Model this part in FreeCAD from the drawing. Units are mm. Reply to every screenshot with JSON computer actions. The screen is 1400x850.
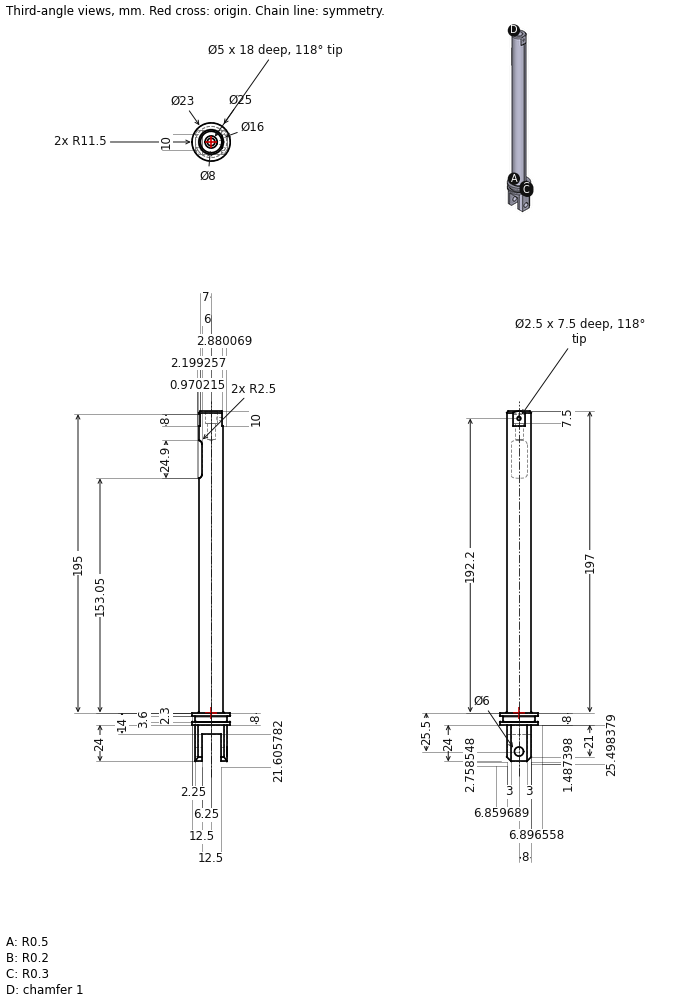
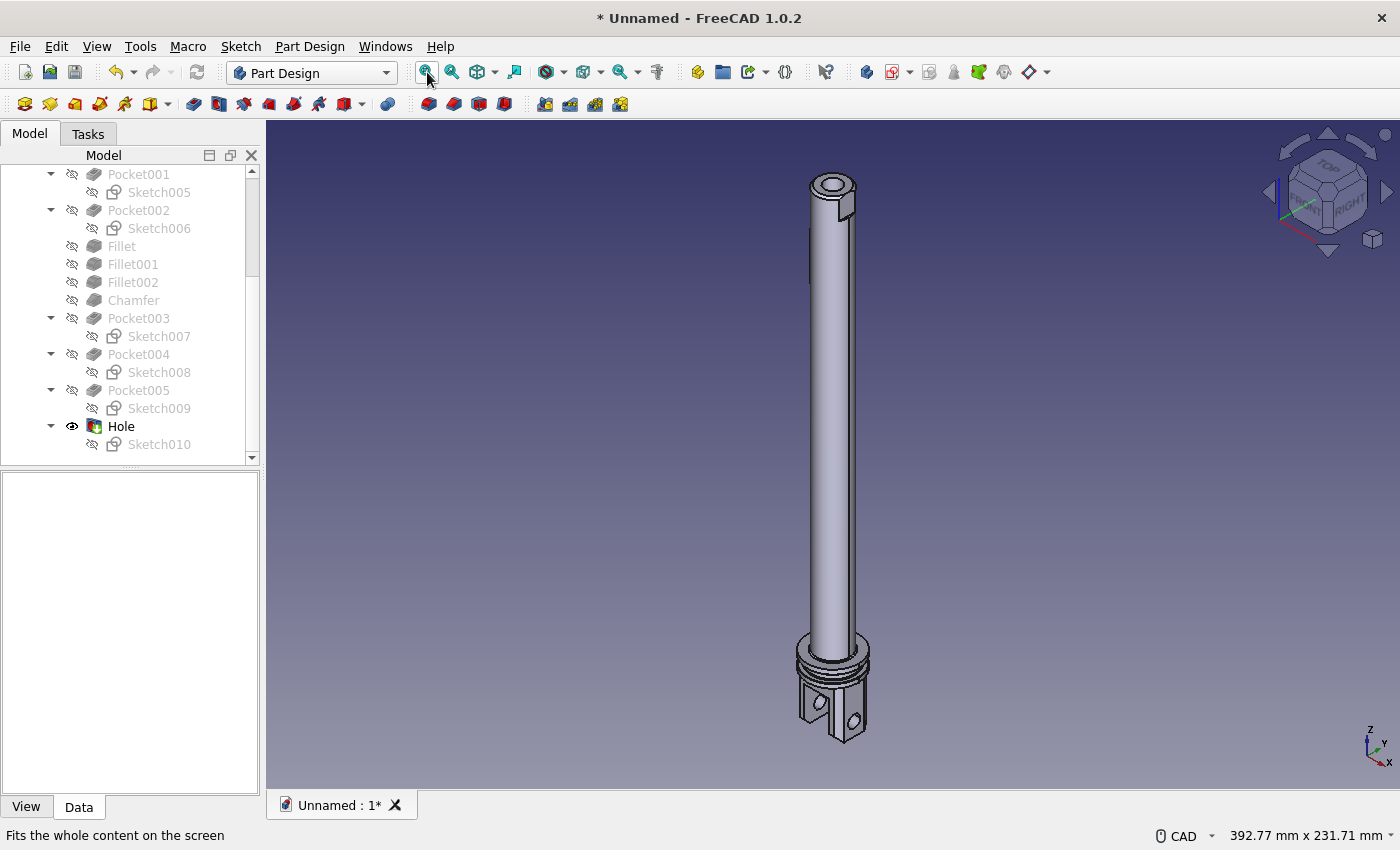
{"action": "left_click", "coordinate": [850, 202]}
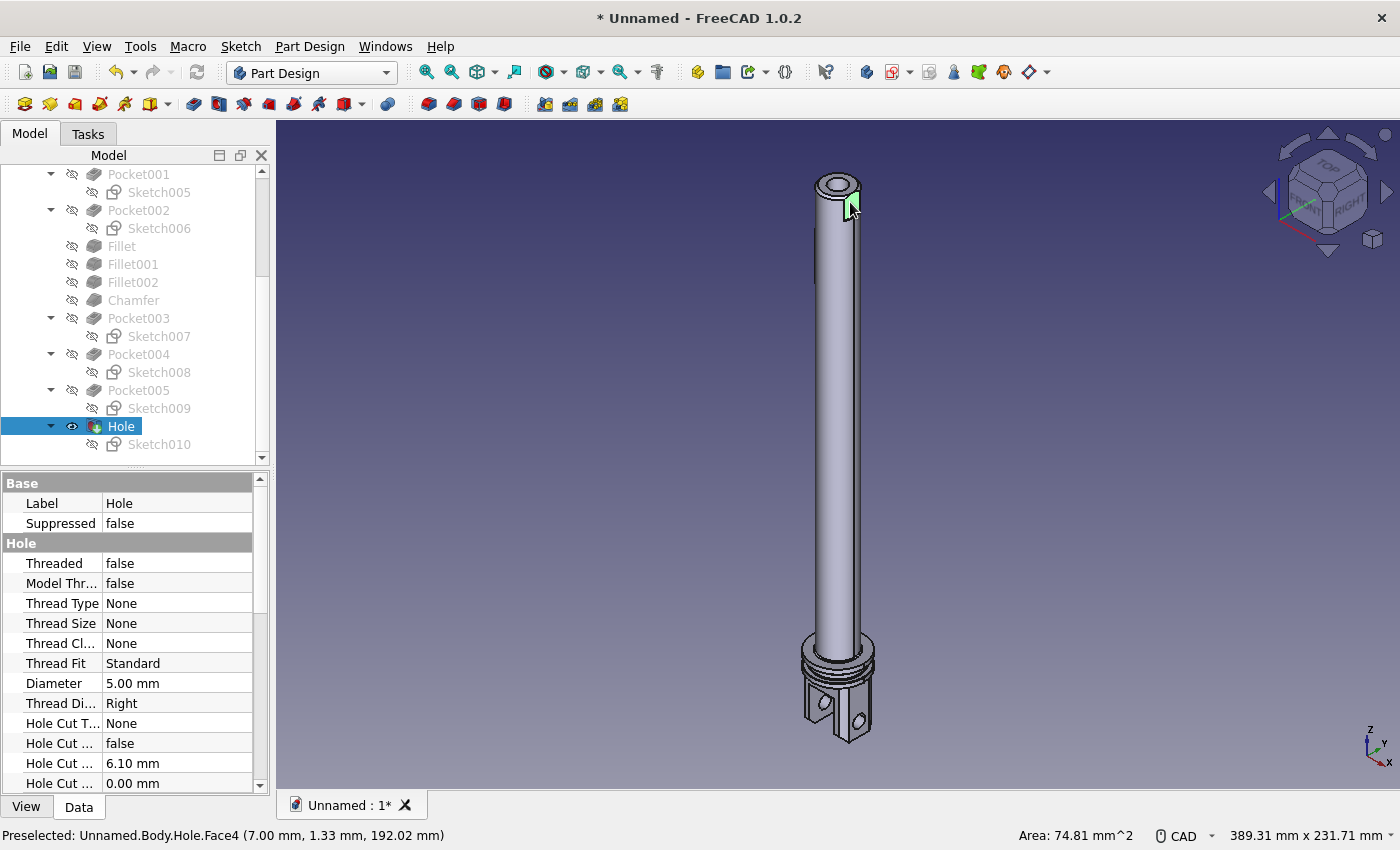
{"action": "left_click", "coordinate": [892, 72]}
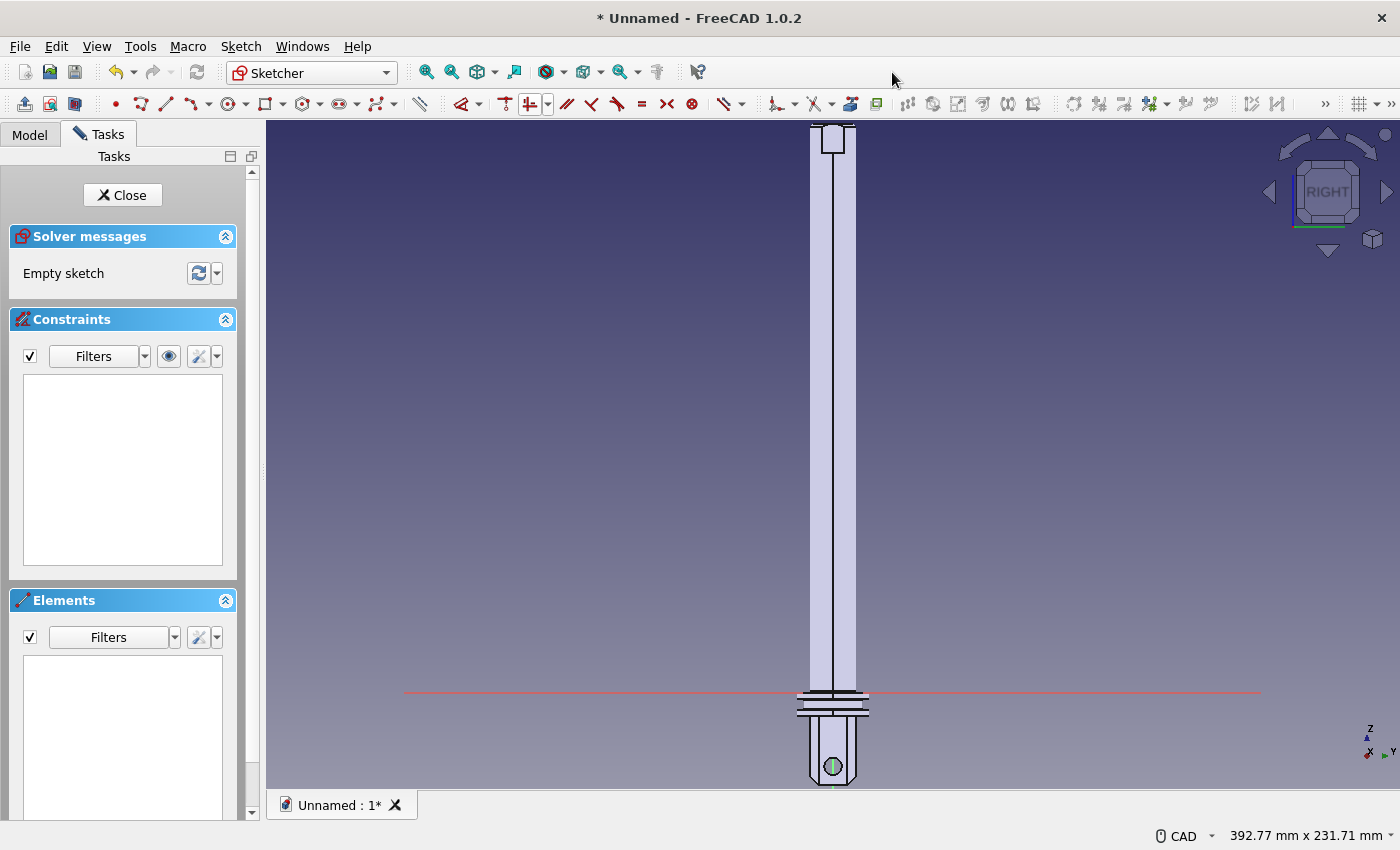
{"action": "left_click", "coordinate": [75, 104]}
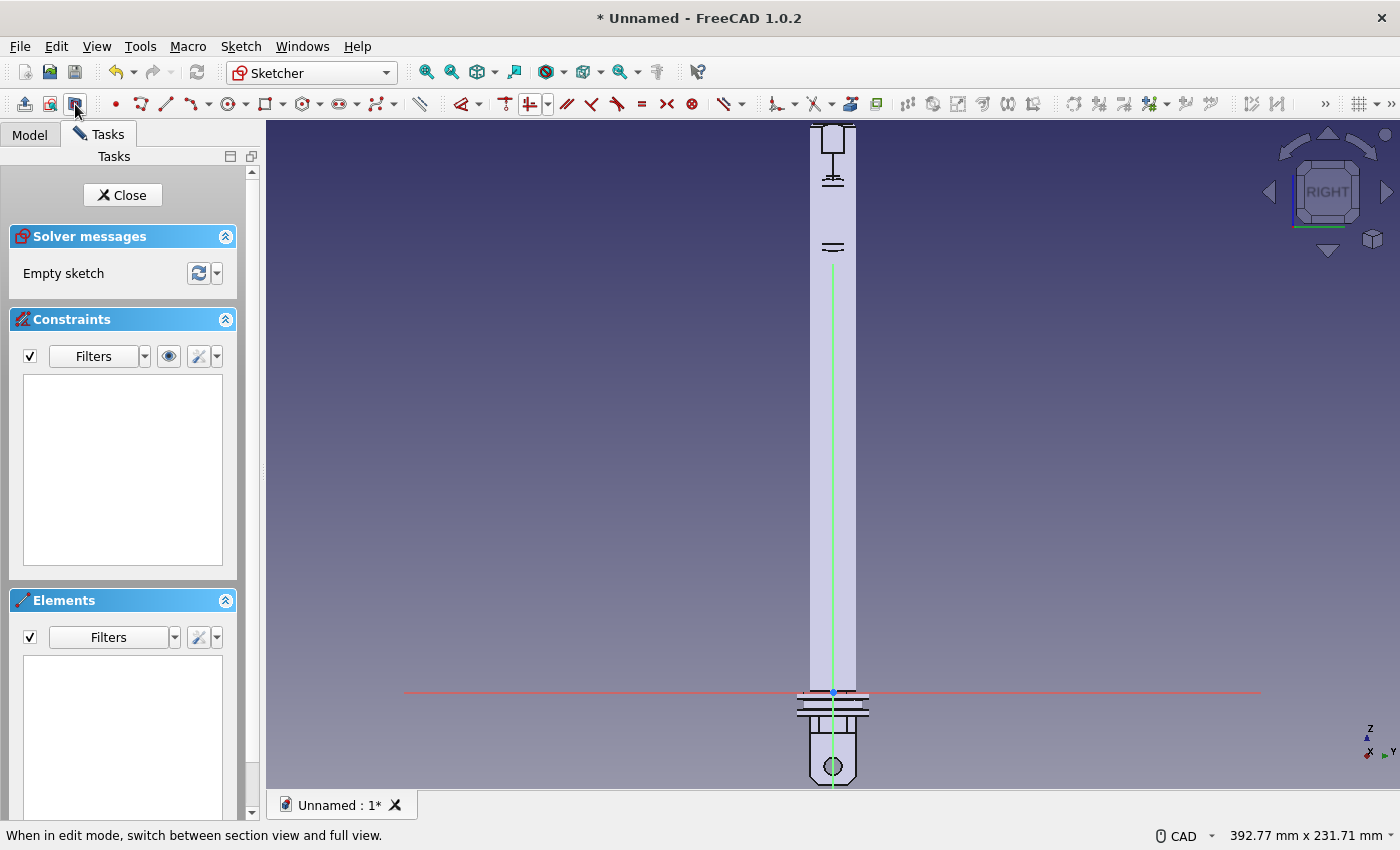
{"action": "scroll", "coordinate": [764, 454], "scroll_direction": "down", "scroll_amount": 5}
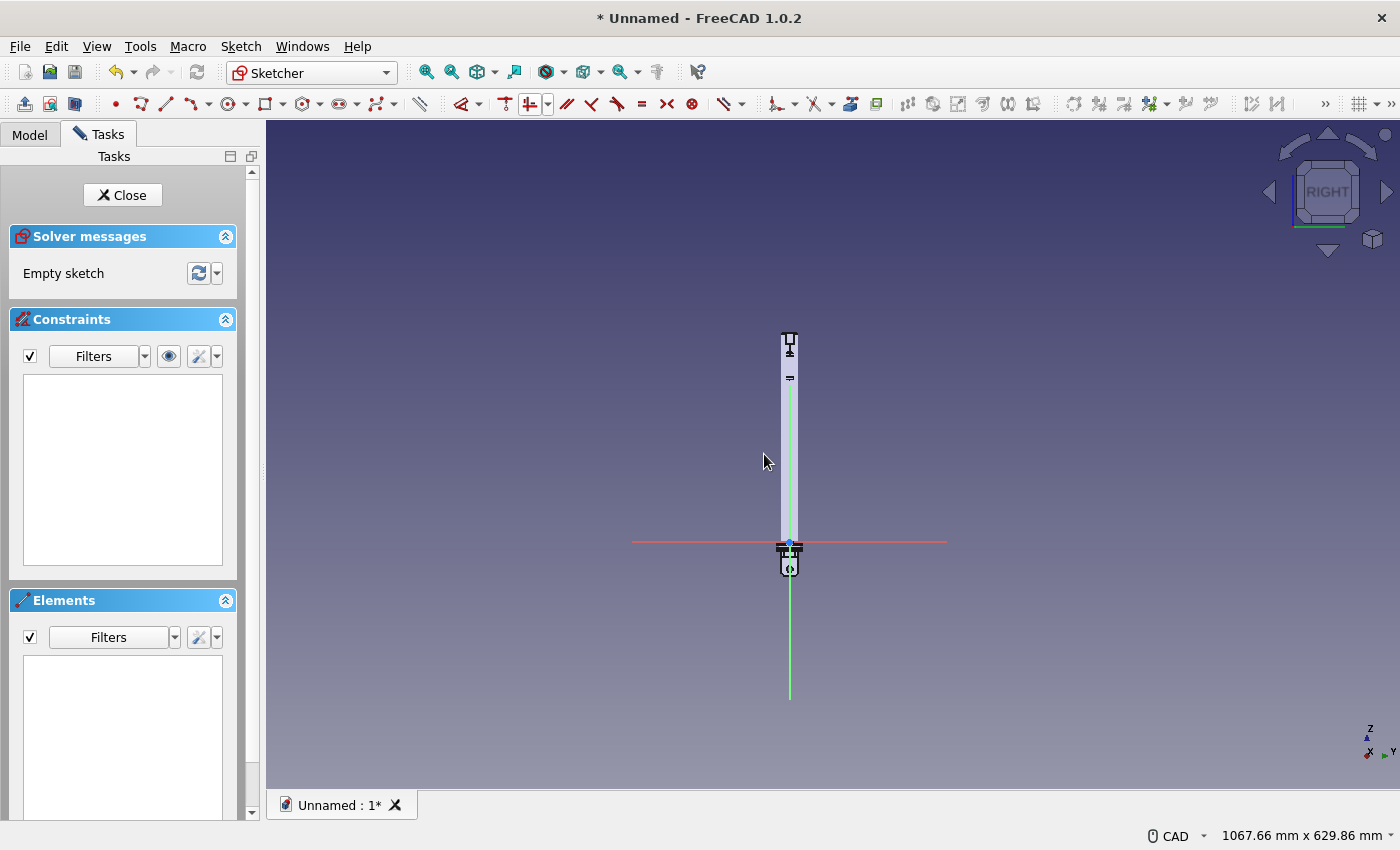
{"action": "scroll", "coordinate": [791, 332], "scroll_direction": "up", "scroll_amount": 15}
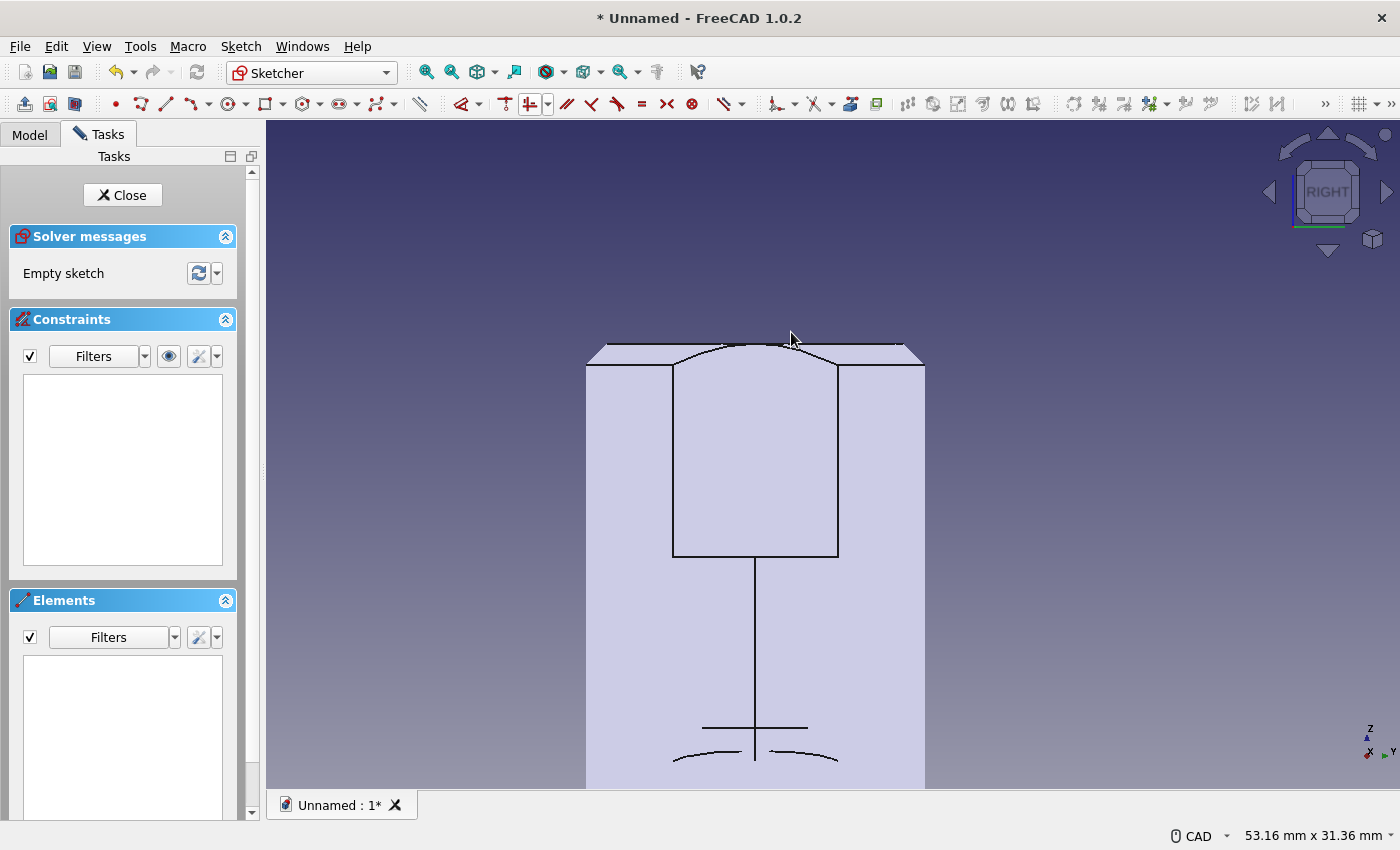
{"action": "scroll", "coordinate": [754, 445], "scroll_direction": "up", "scroll_amount": 10}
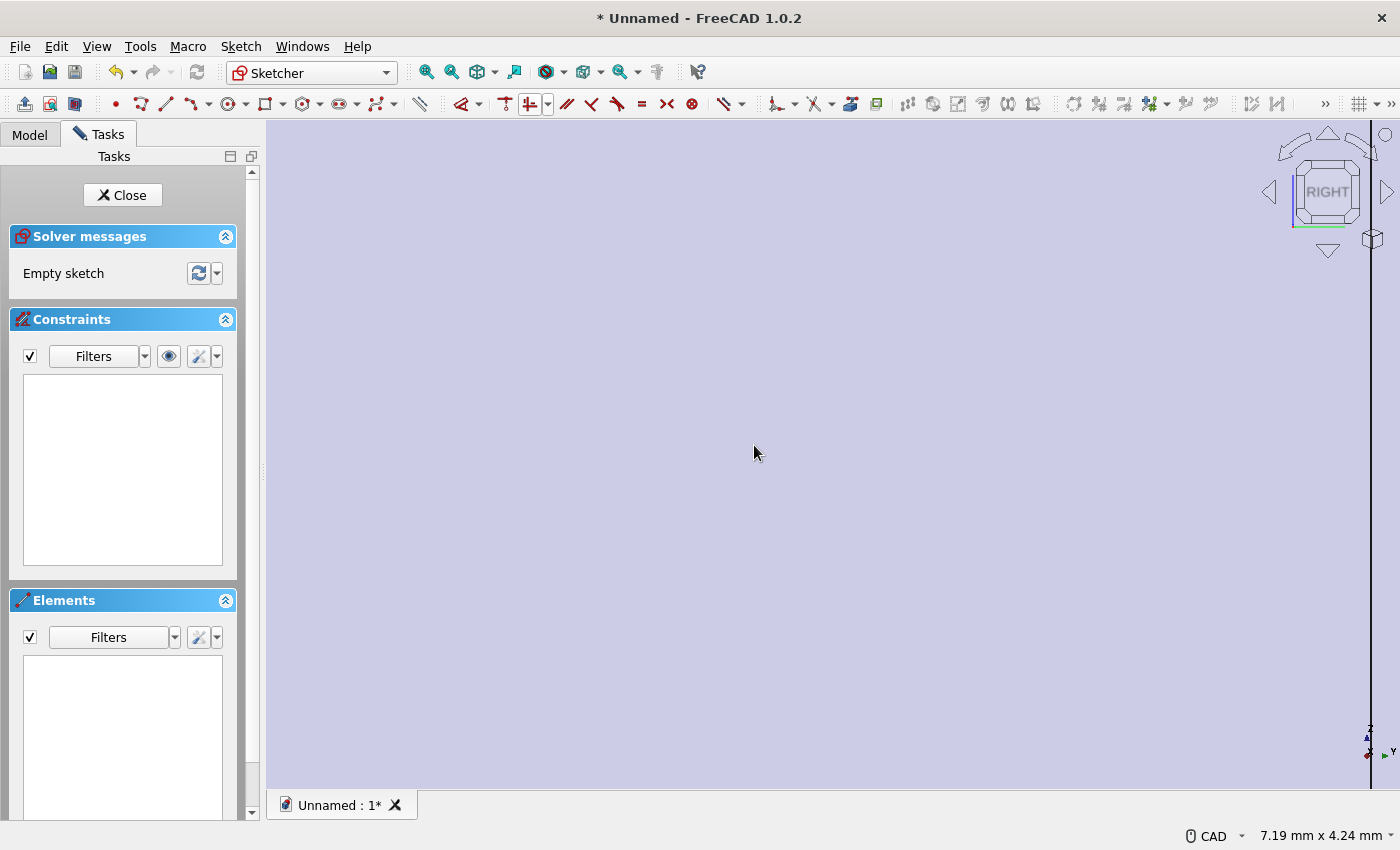
{"action": "left_click", "coordinate": [228, 104]}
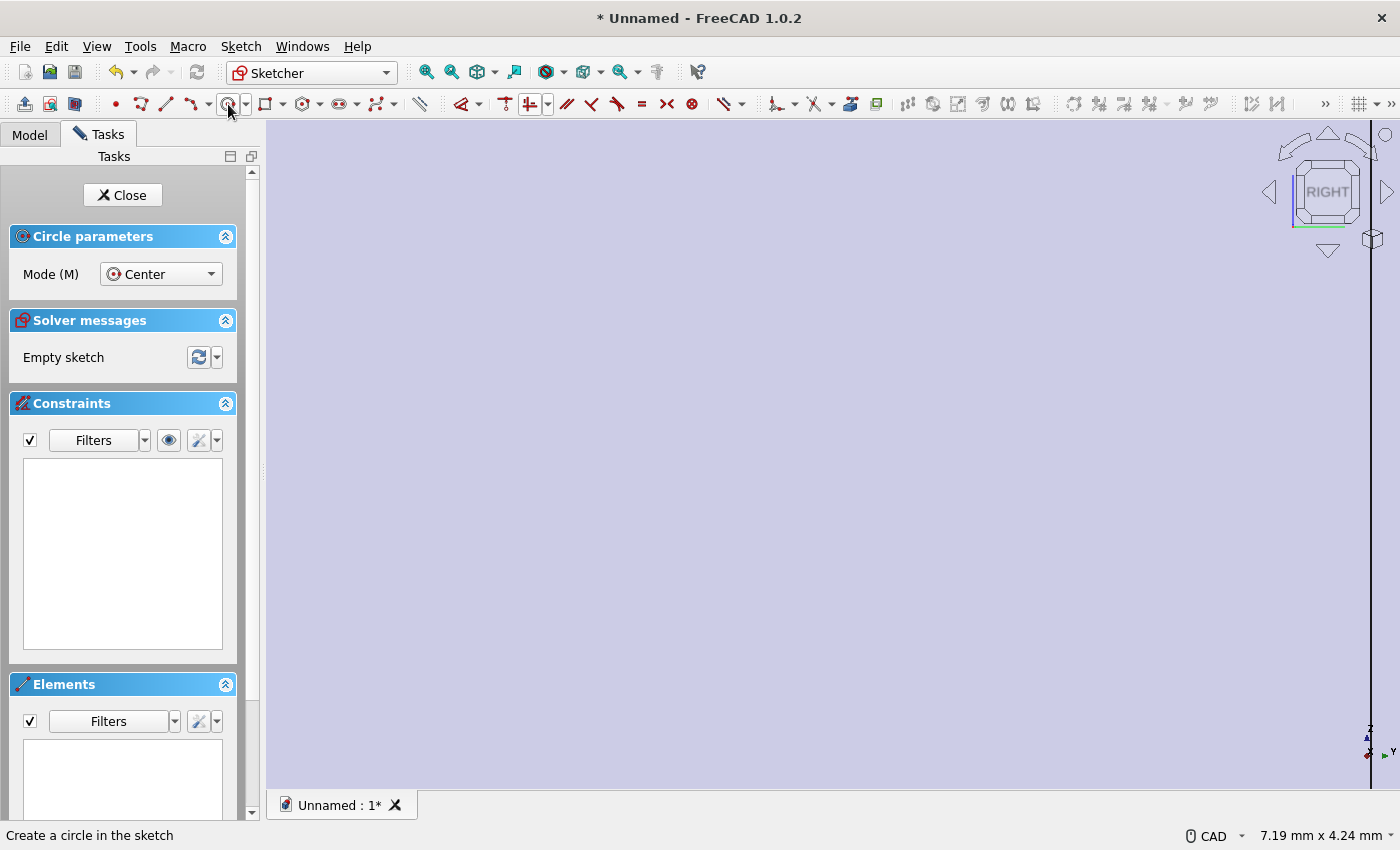
{"action": "left_click", "coordinate": [761, 450]}
{"action": "mouse_move", "coordinate": [900, 311]}